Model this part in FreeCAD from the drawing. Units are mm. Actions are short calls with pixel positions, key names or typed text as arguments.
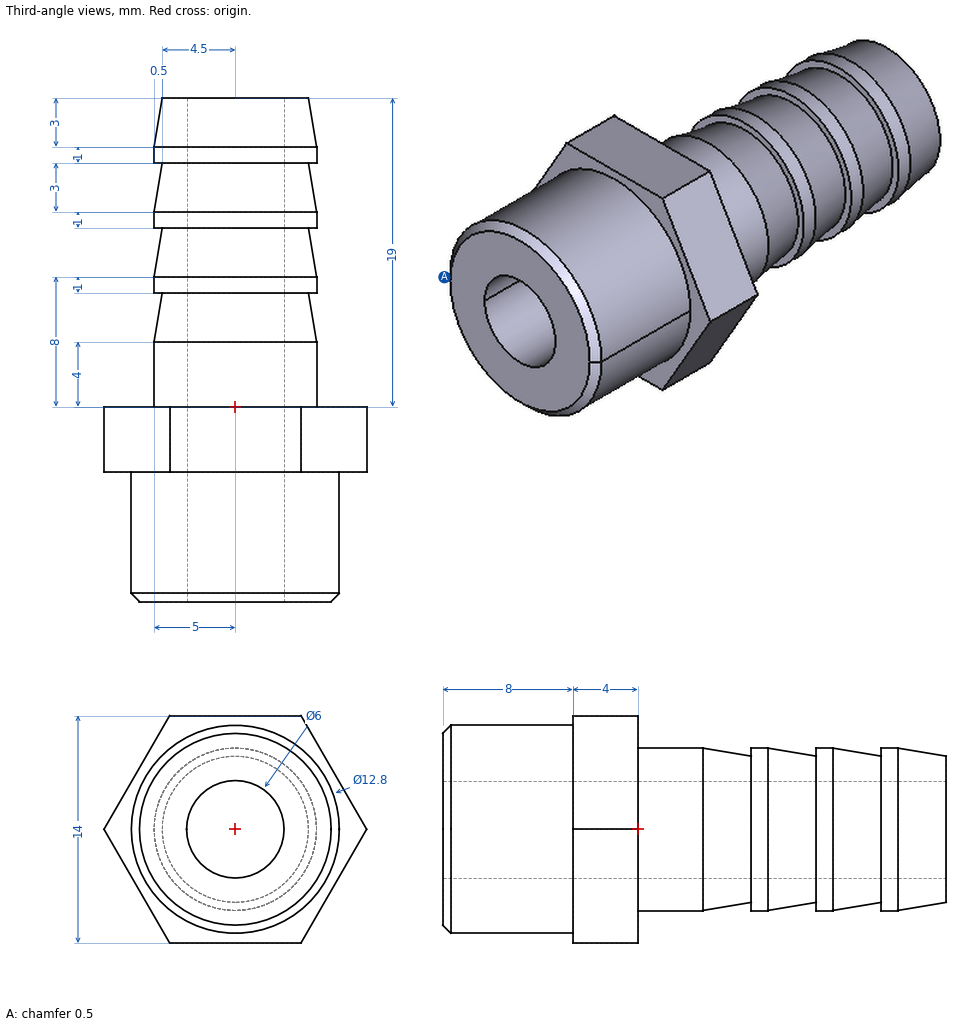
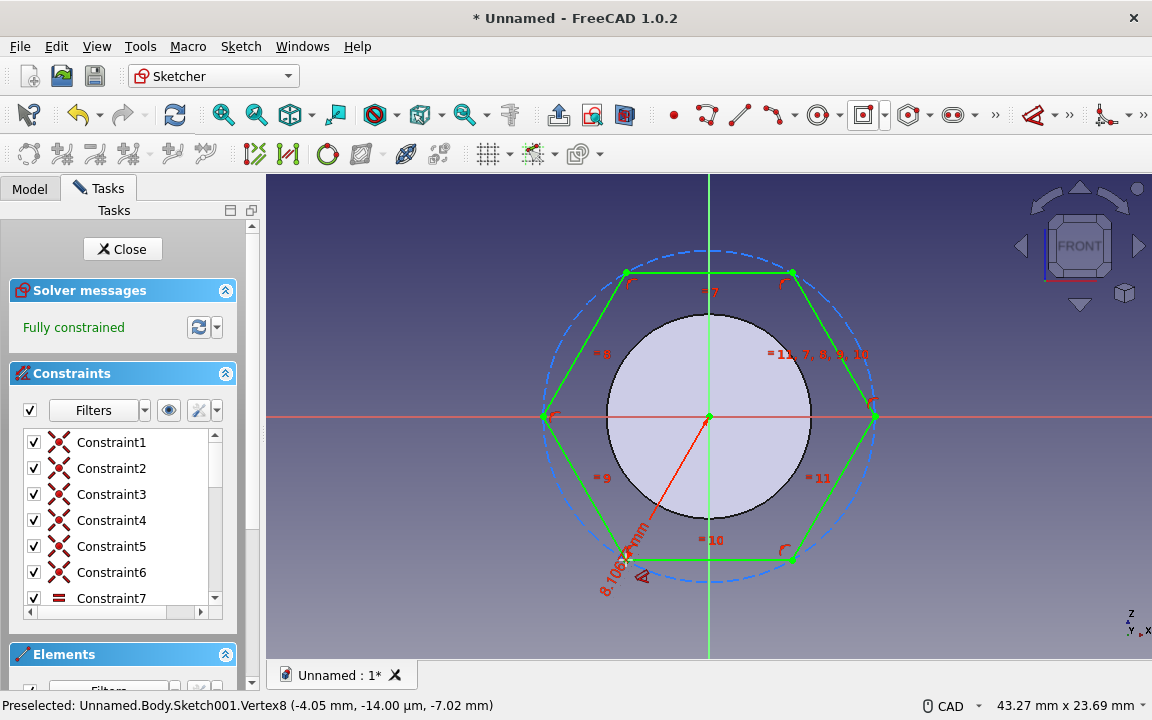
click(792, 273)
click(874, 316)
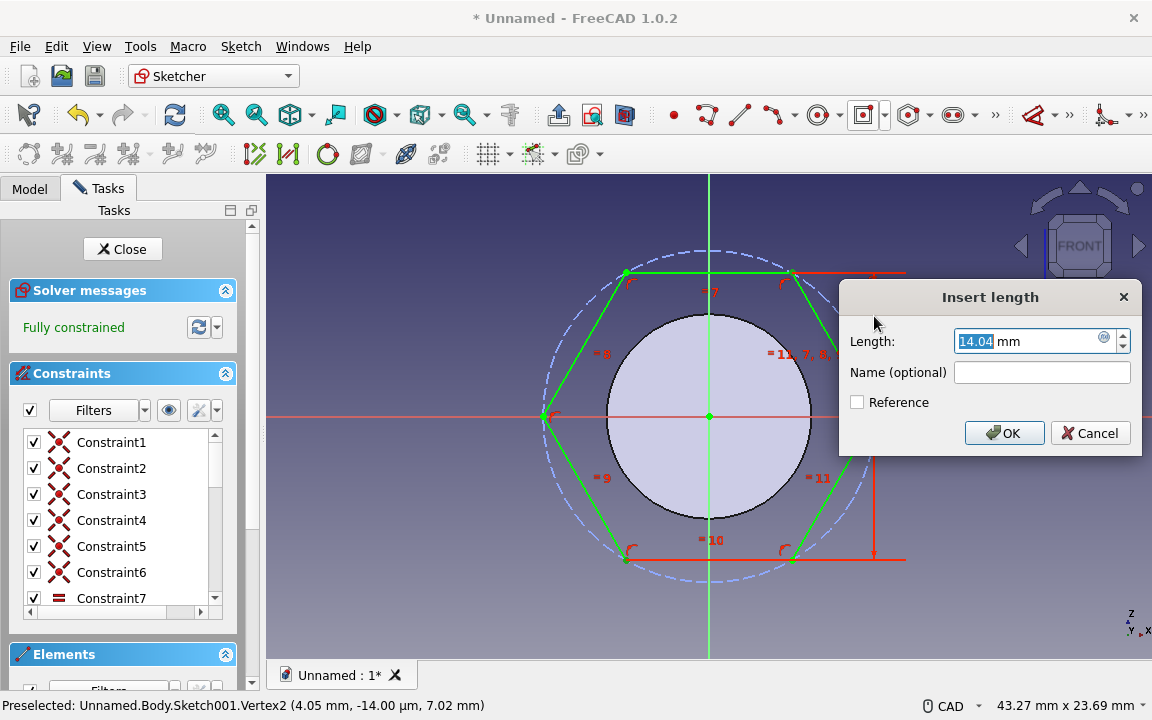
text(14)
key(Return)
key(Escape)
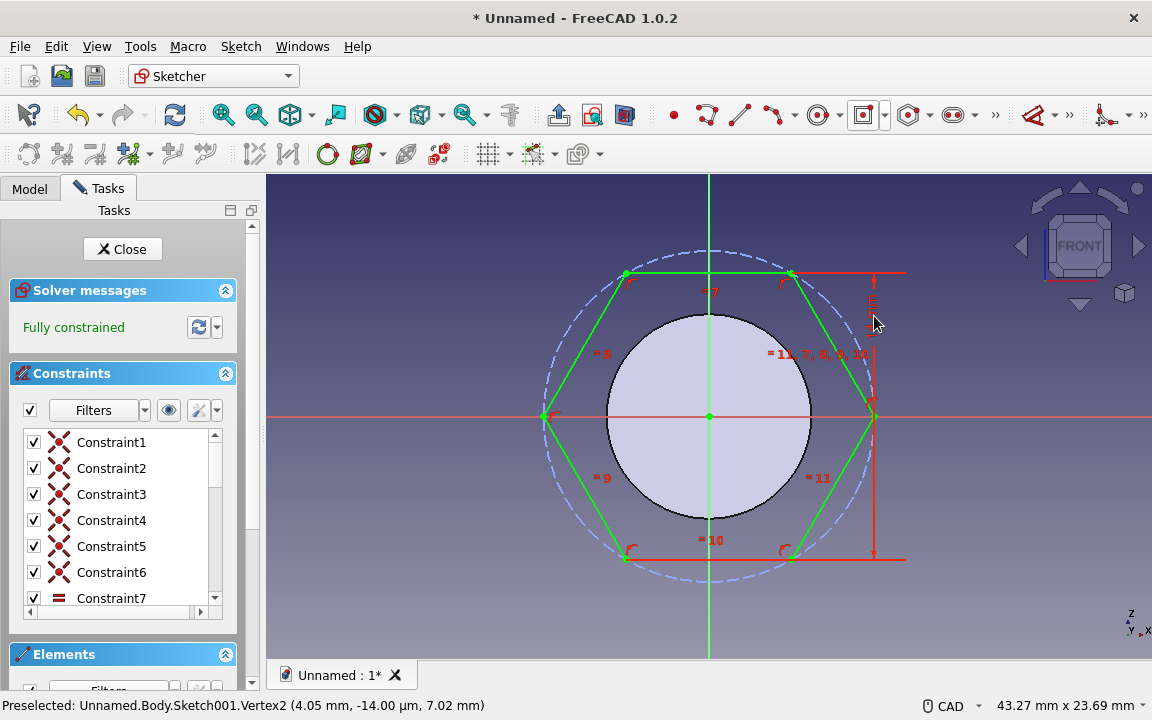
click(123, 249)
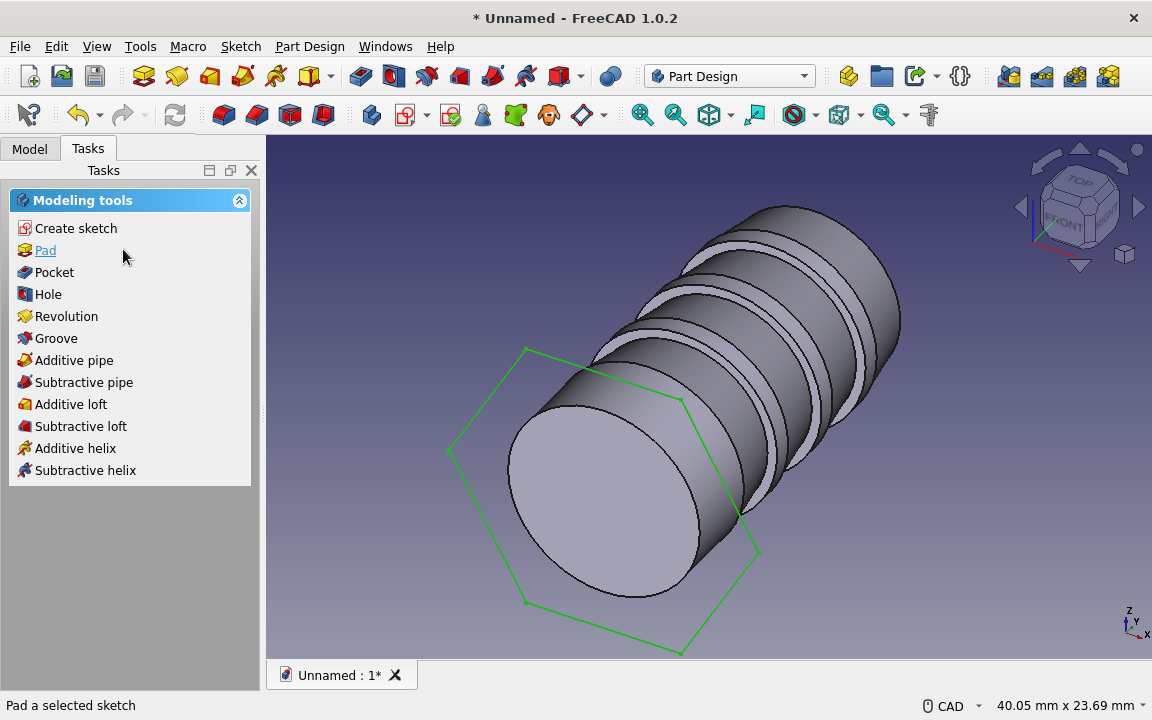
click(144, 76)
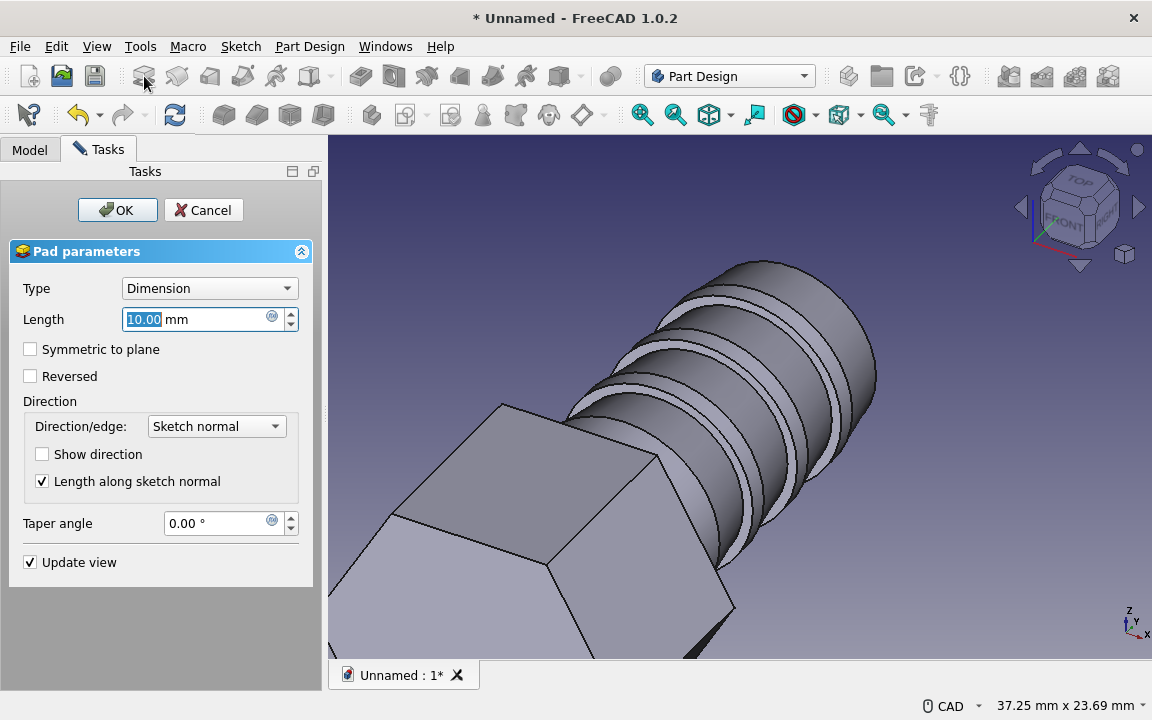
text(4)
key(Tab)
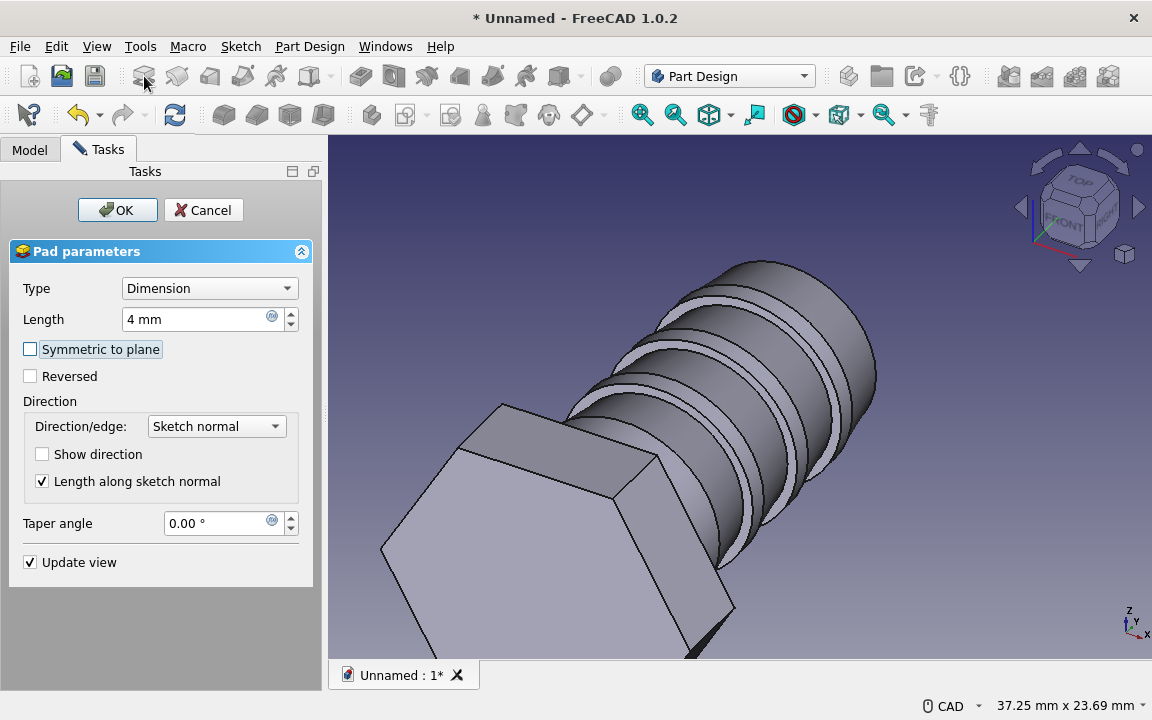
click(118, 210)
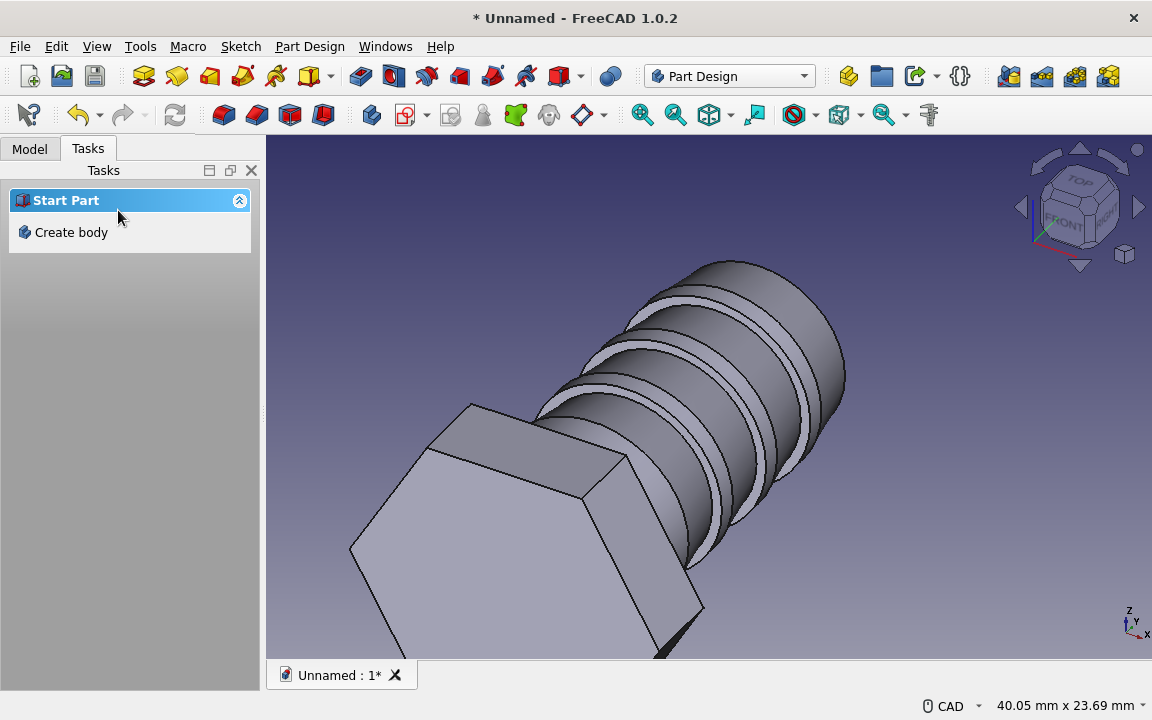
click(643, 116)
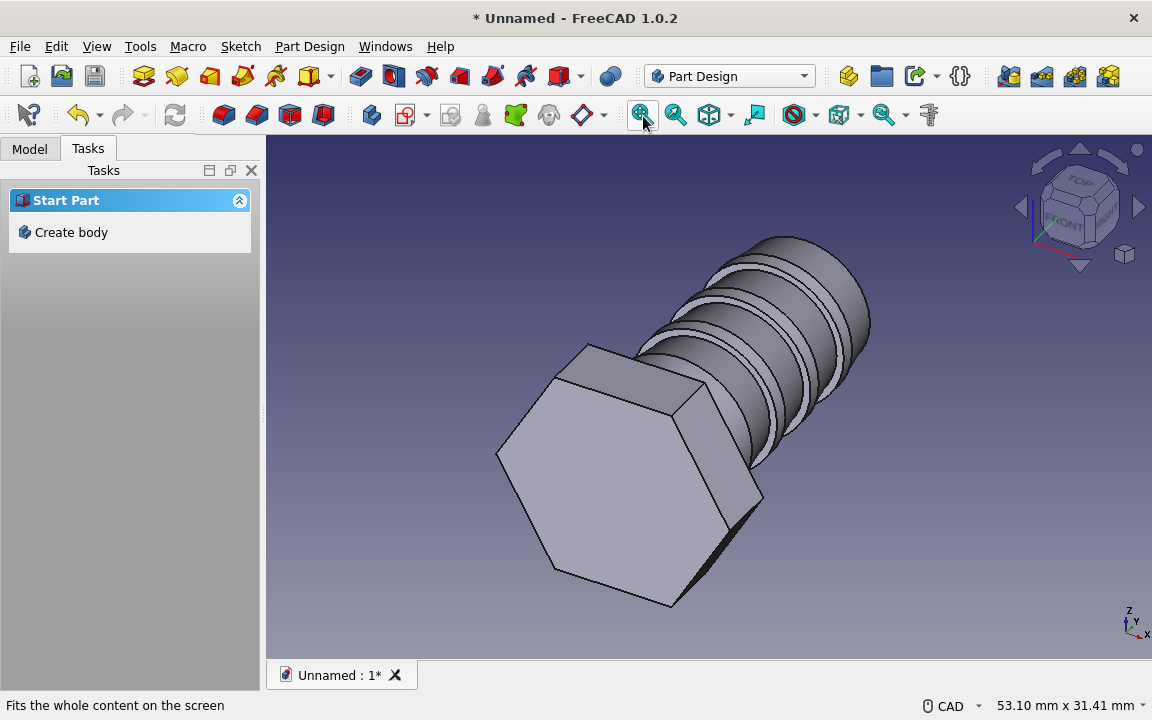
click(613, 491)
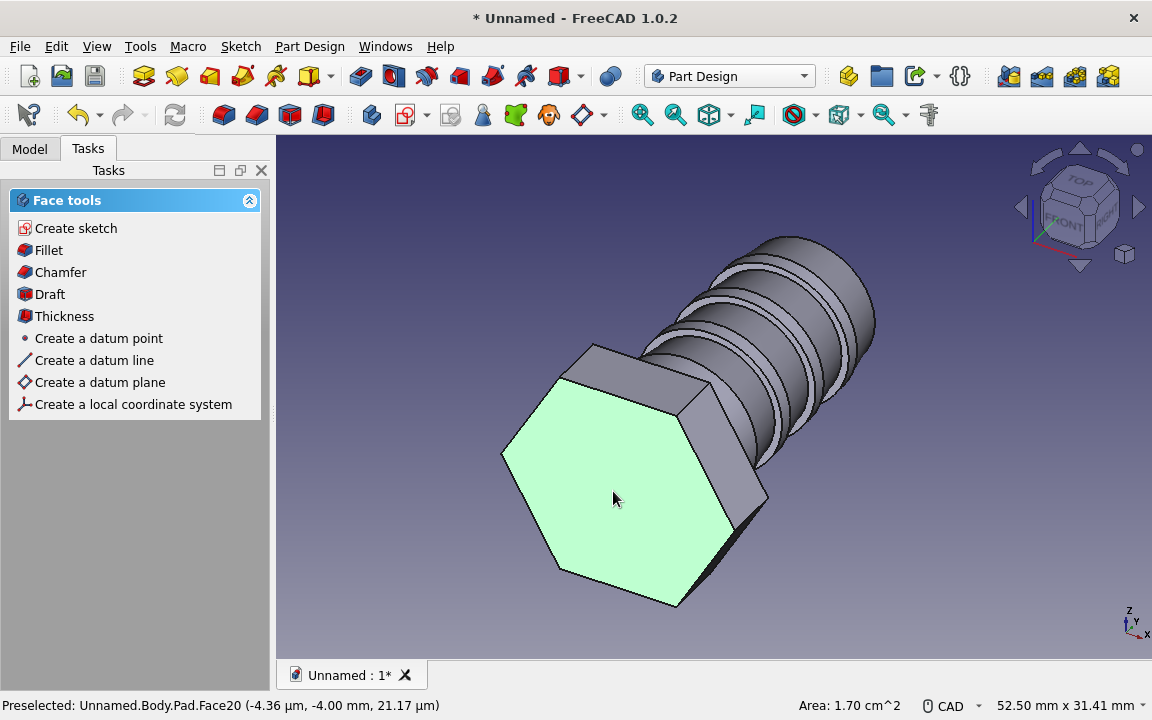
click(404, 116)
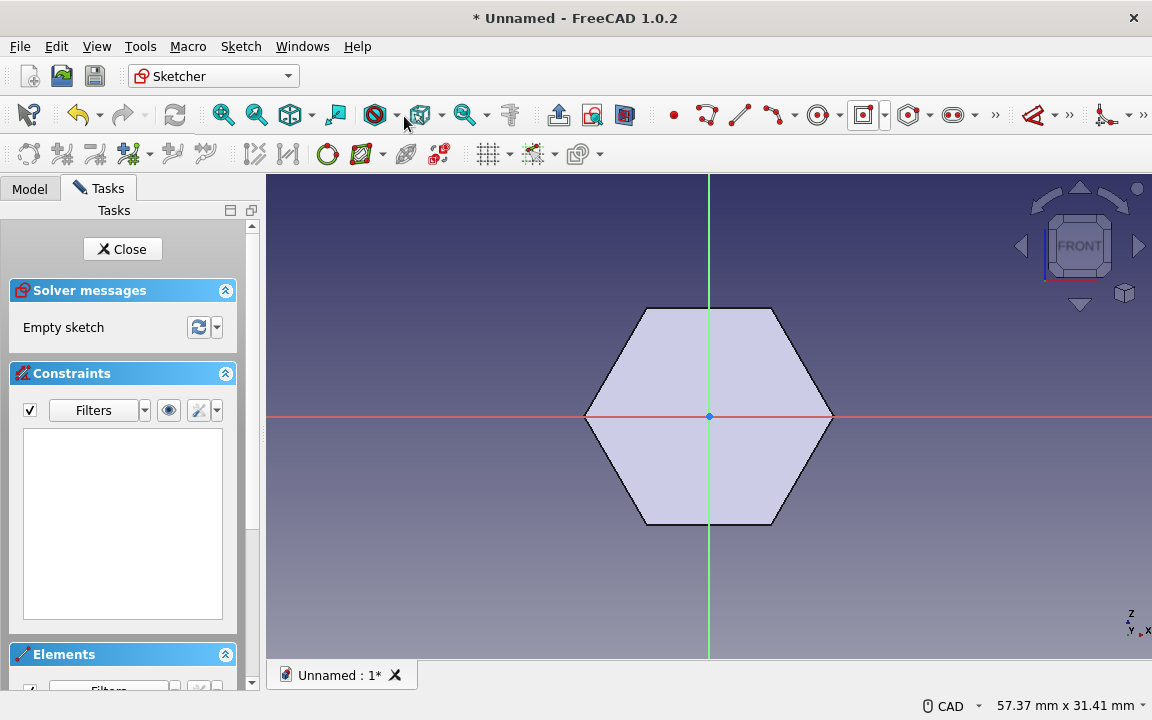
scroll(848, 417, up, 2)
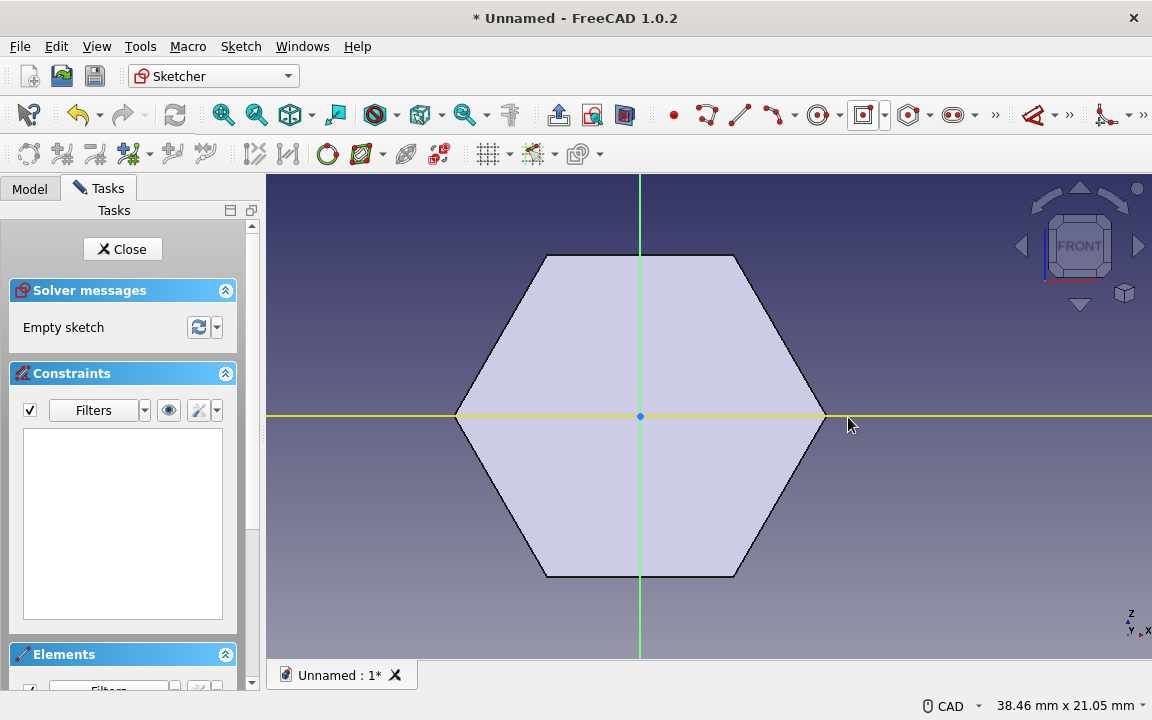
click(818, 116)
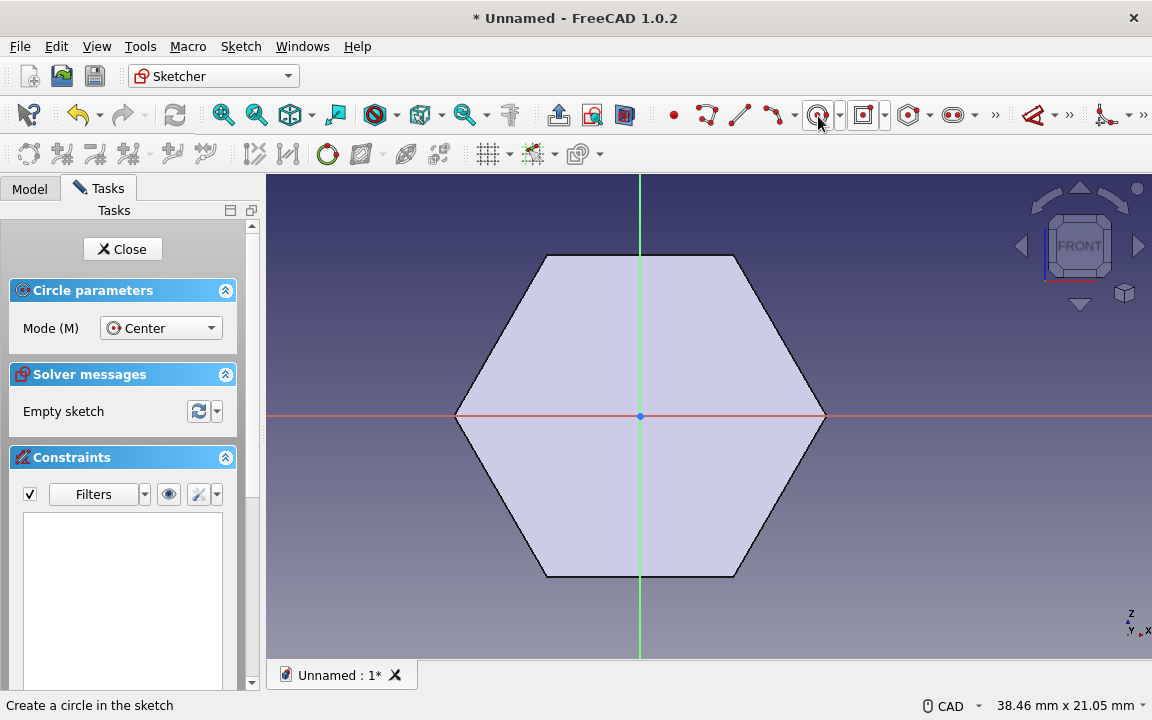
click(640, 416)
click(745, 312)
key(Escape)